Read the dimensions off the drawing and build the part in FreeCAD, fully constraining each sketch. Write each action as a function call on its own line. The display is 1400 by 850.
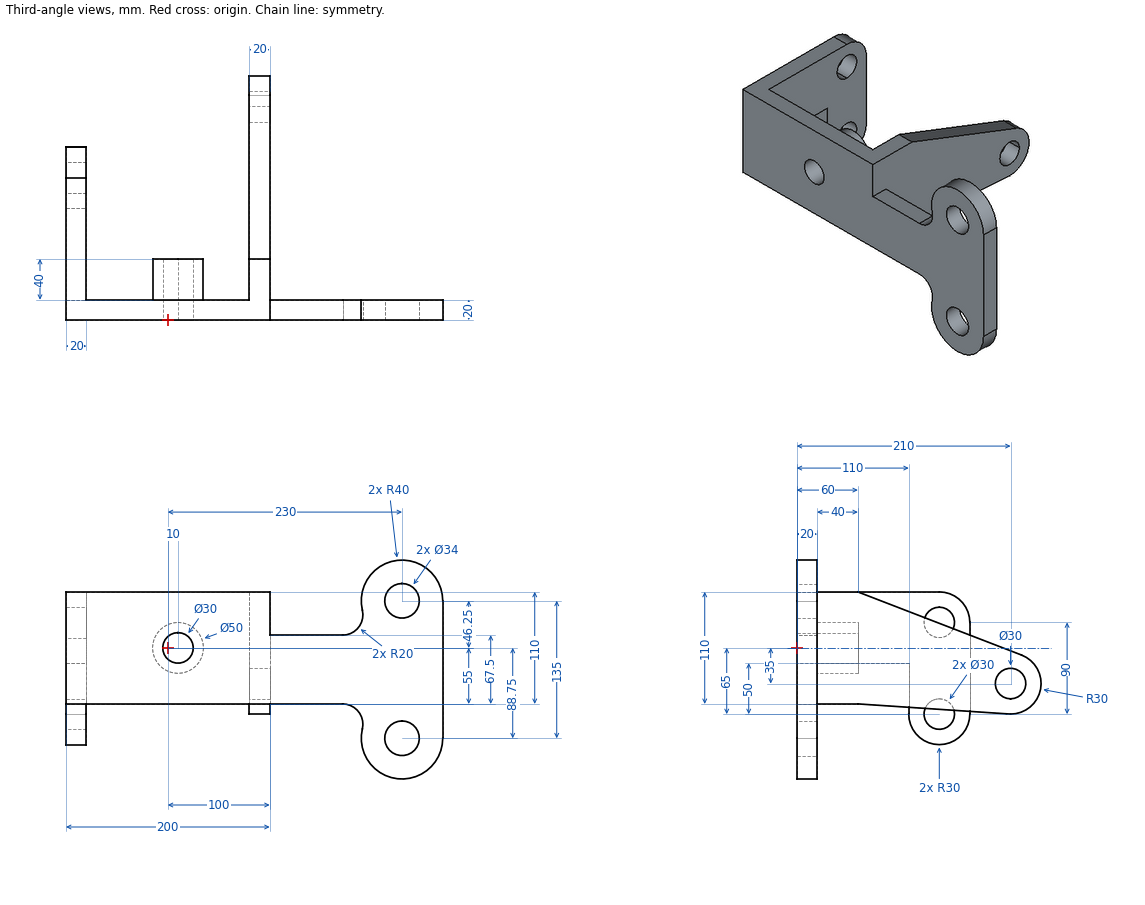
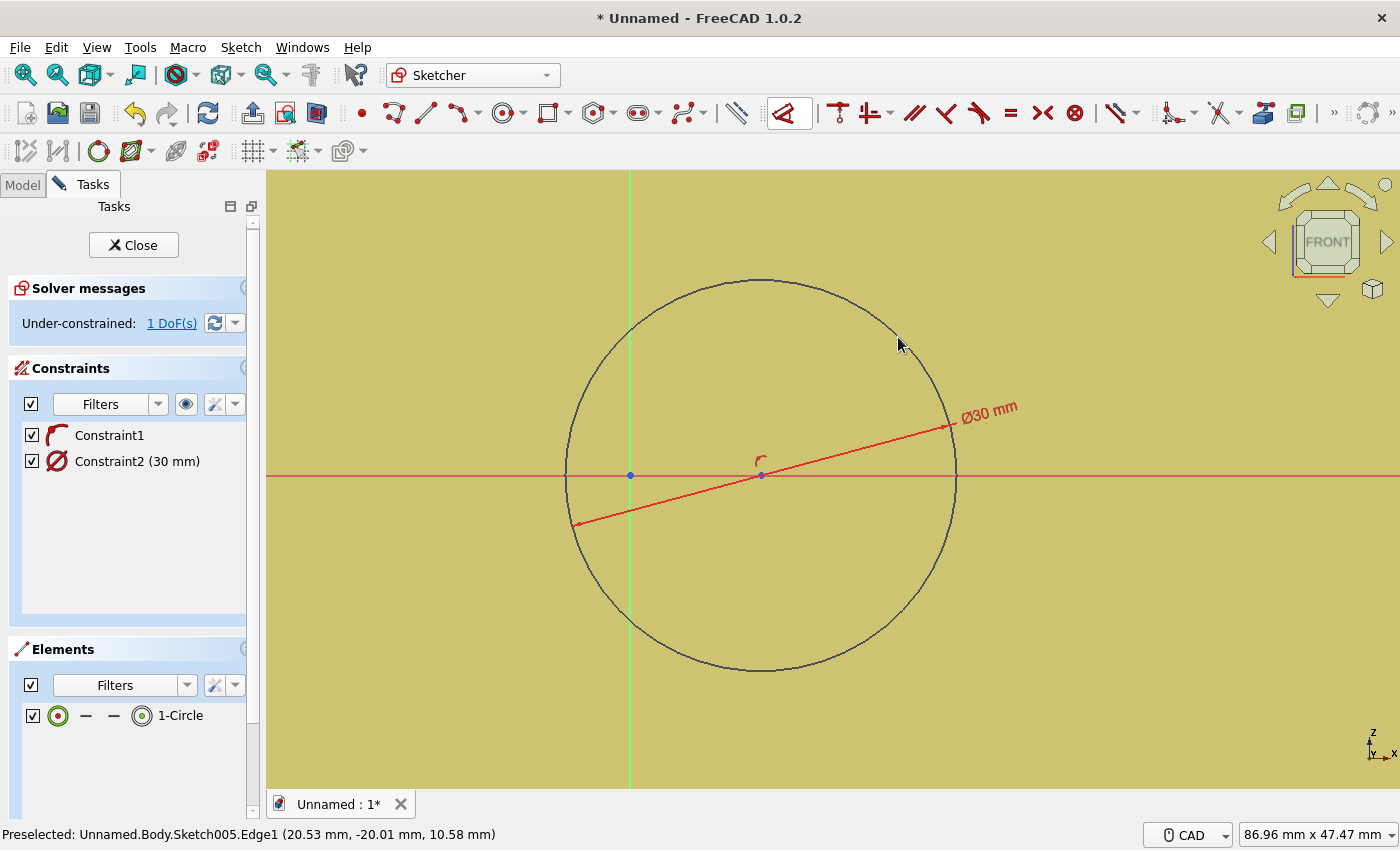
click(761, 476)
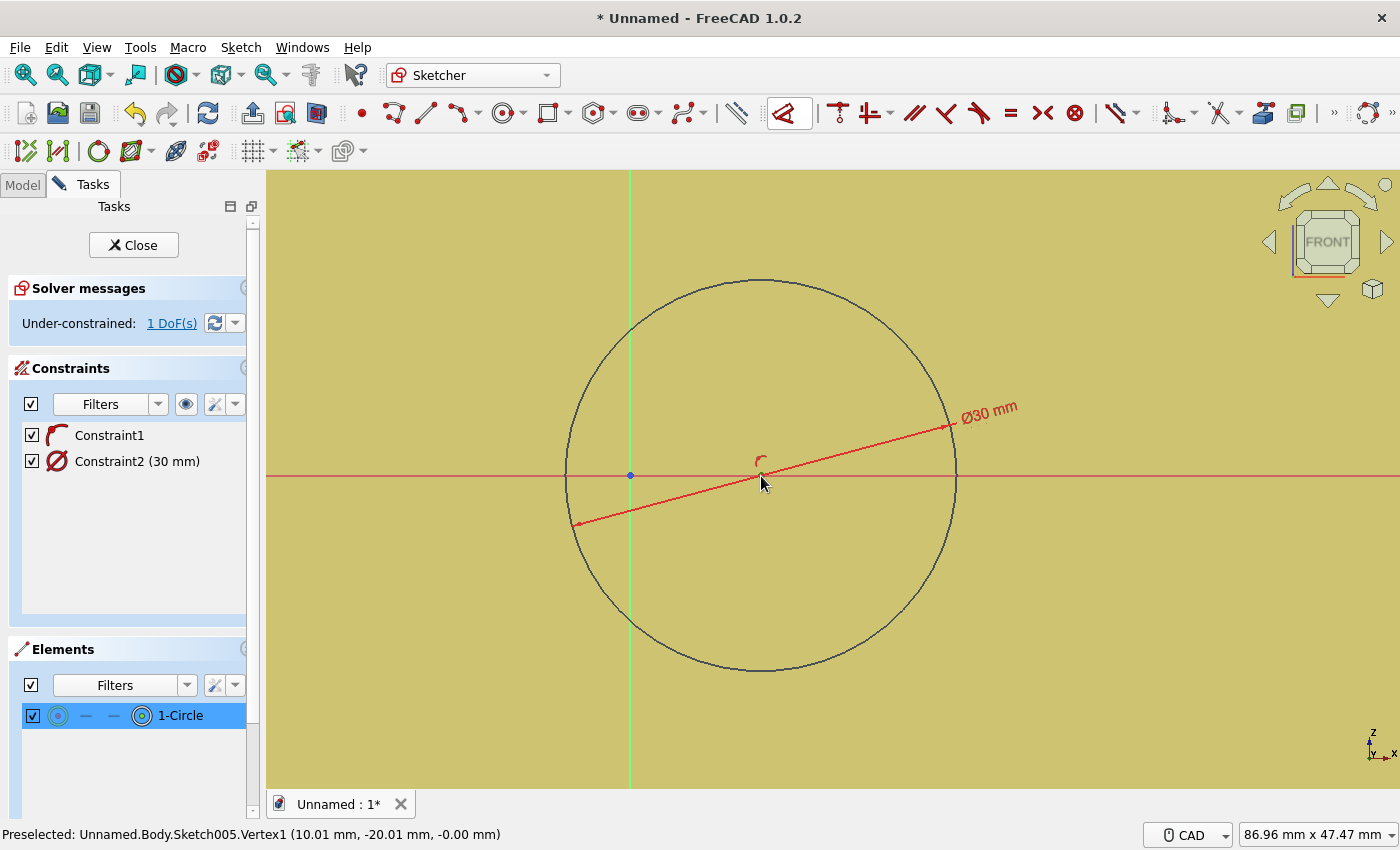
click(806, 114)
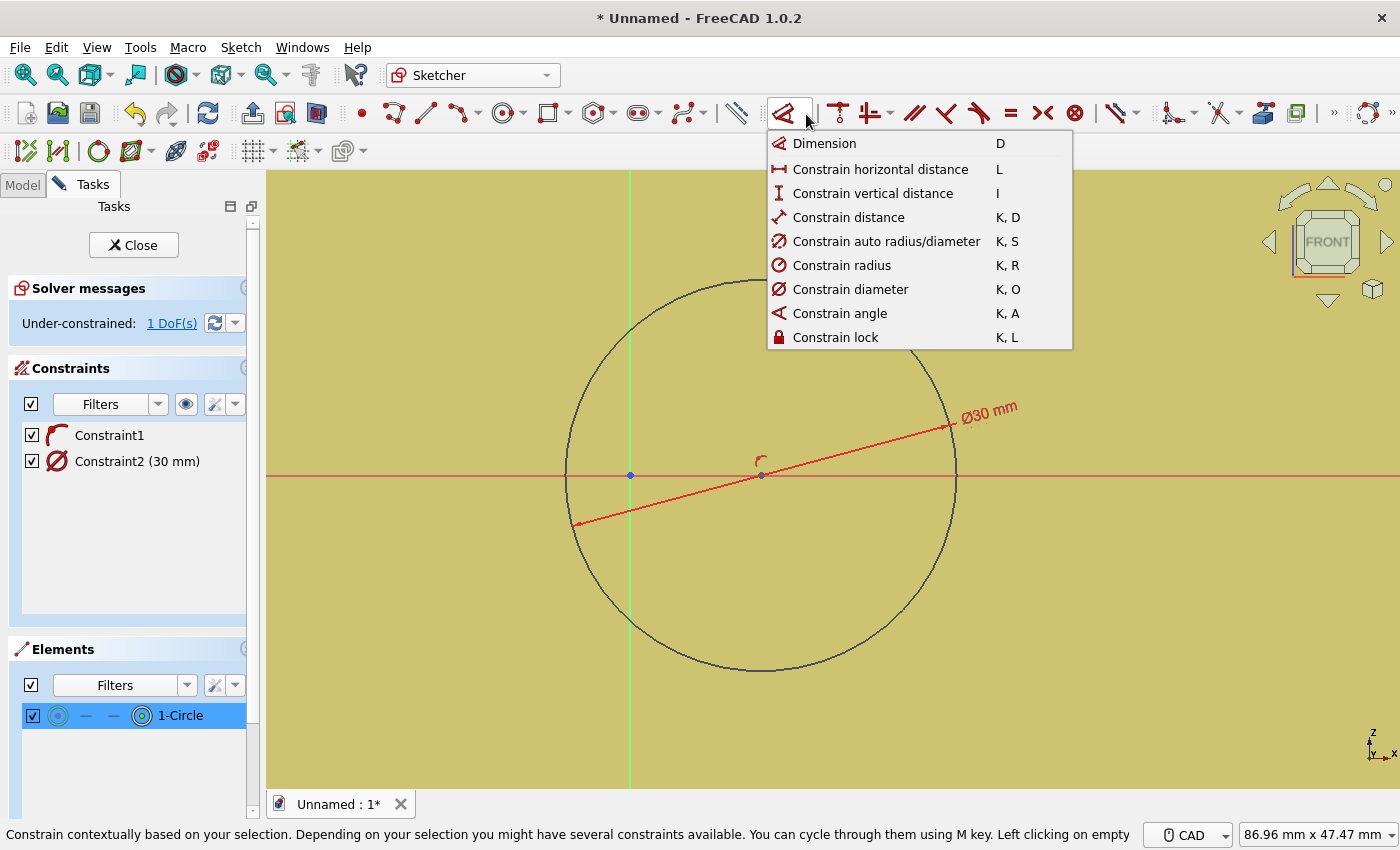
click(920, 169)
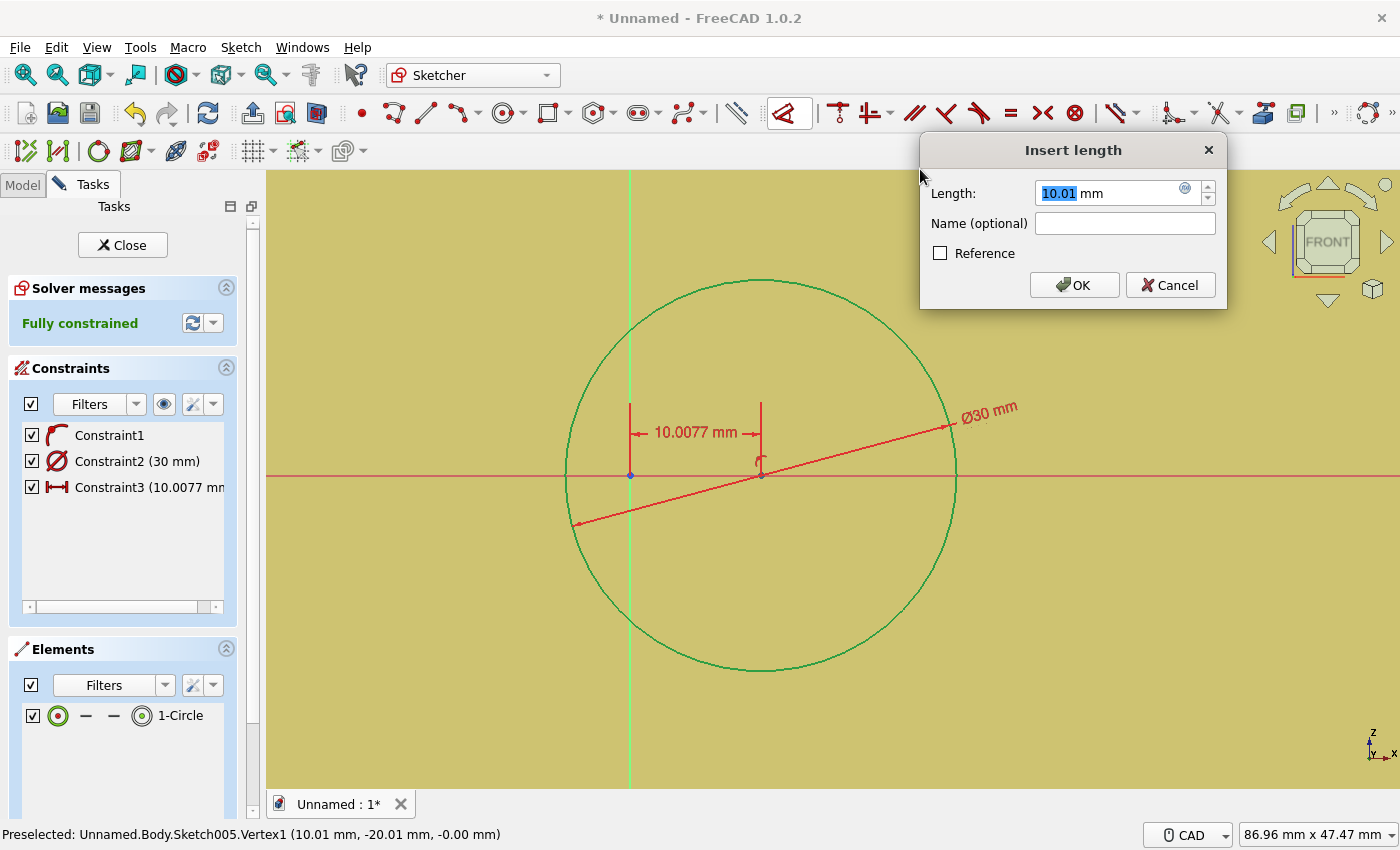
text(10)
key(Return)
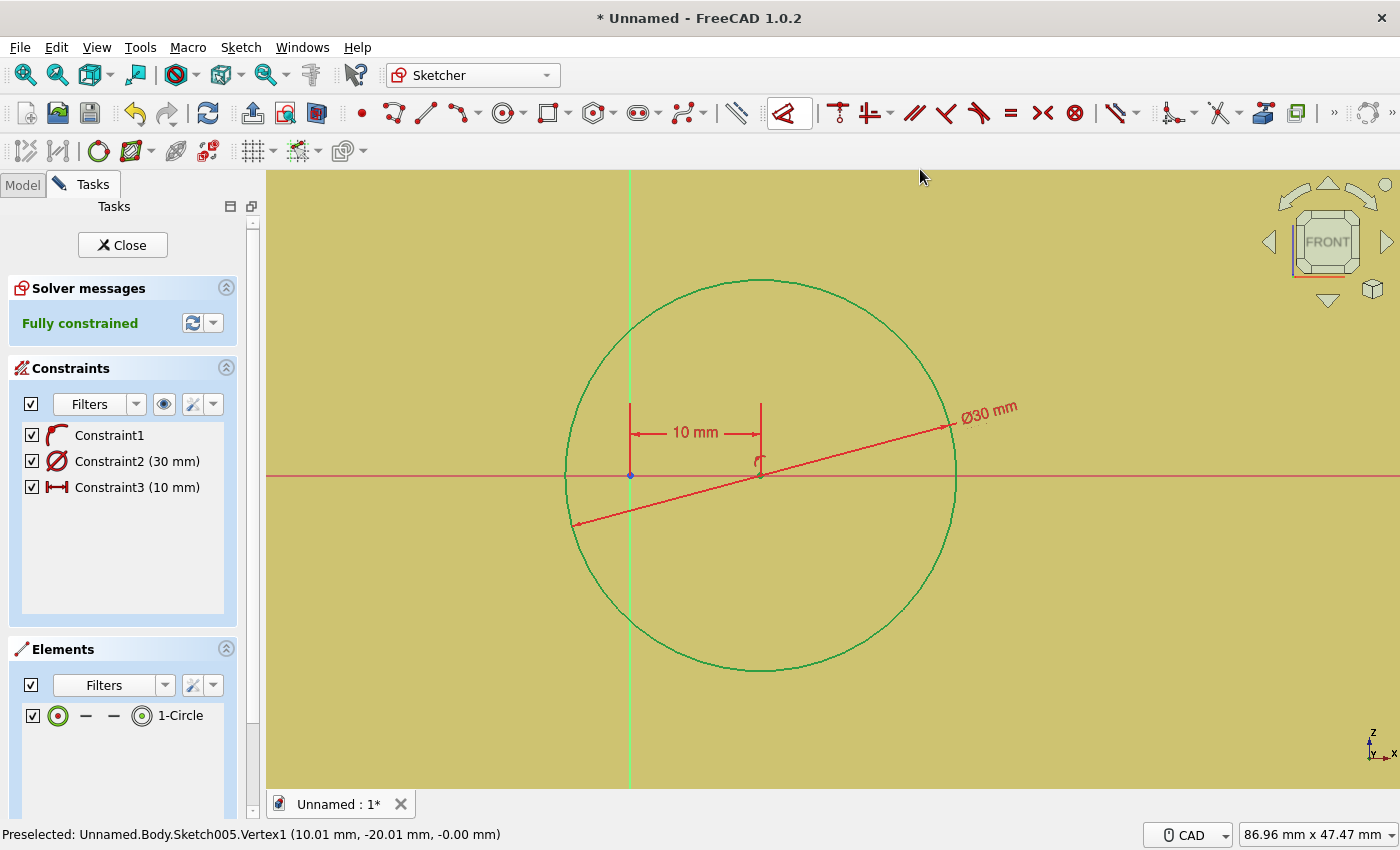
click(123, 245)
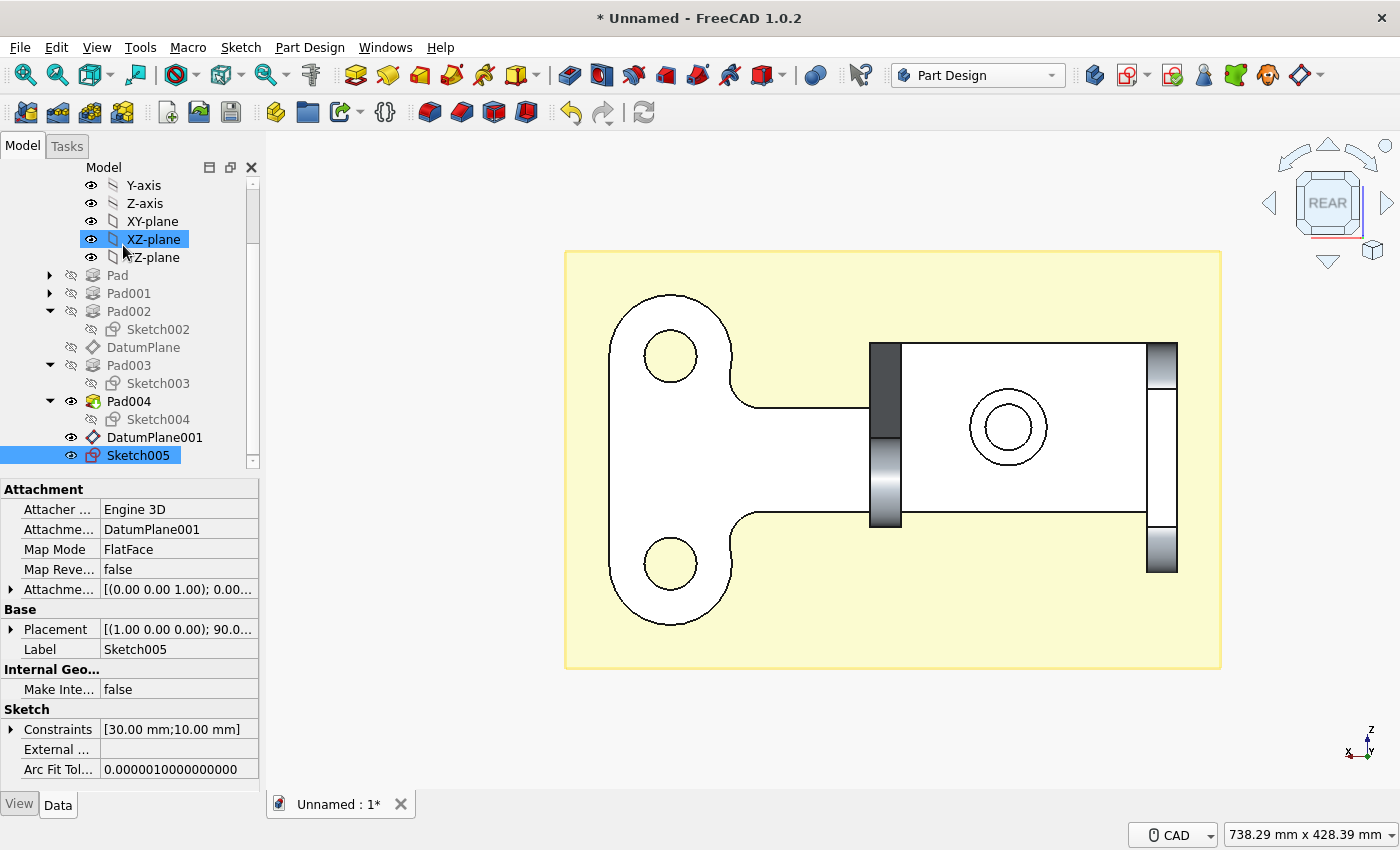
click(570, 76)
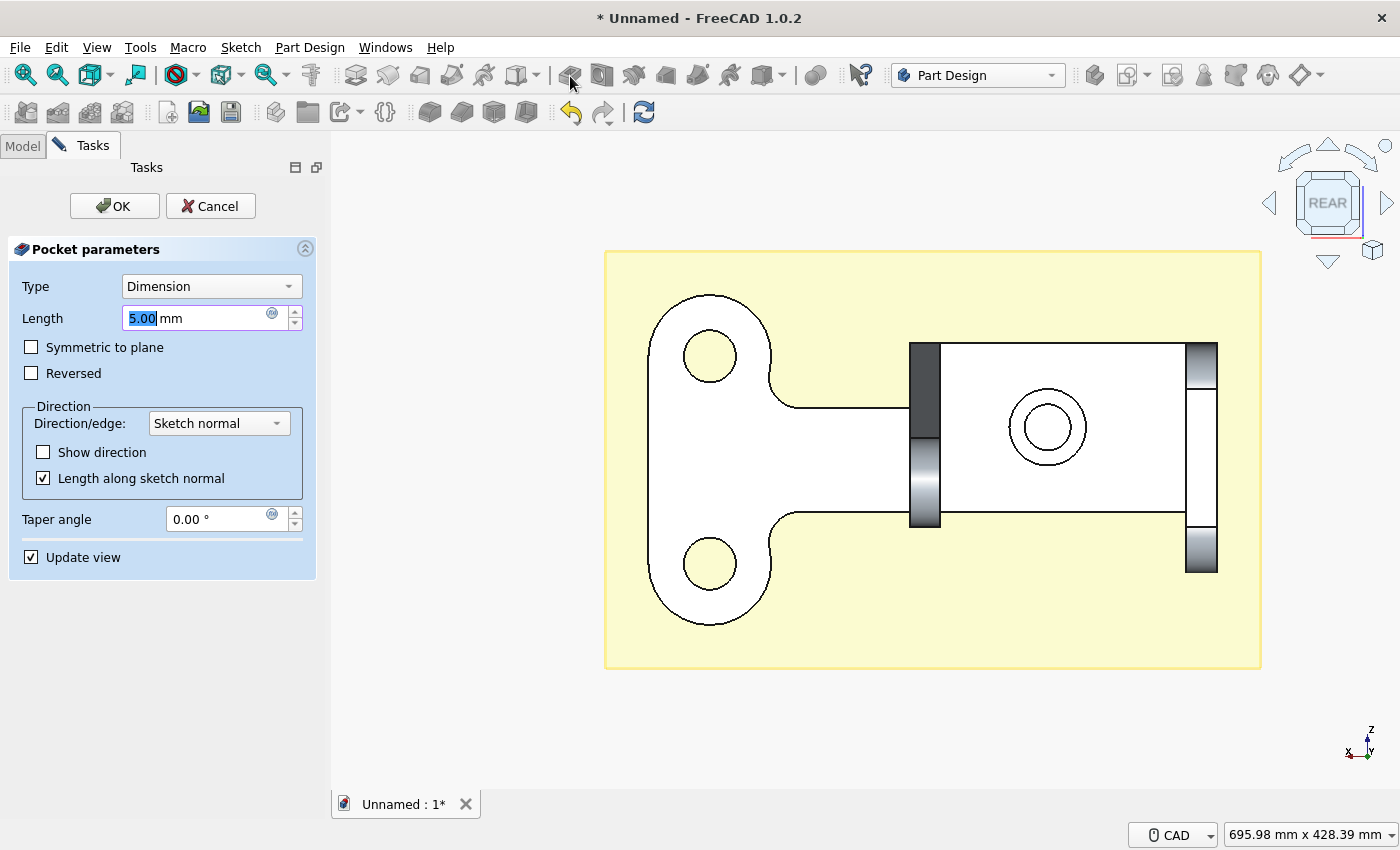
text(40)
key(Tab)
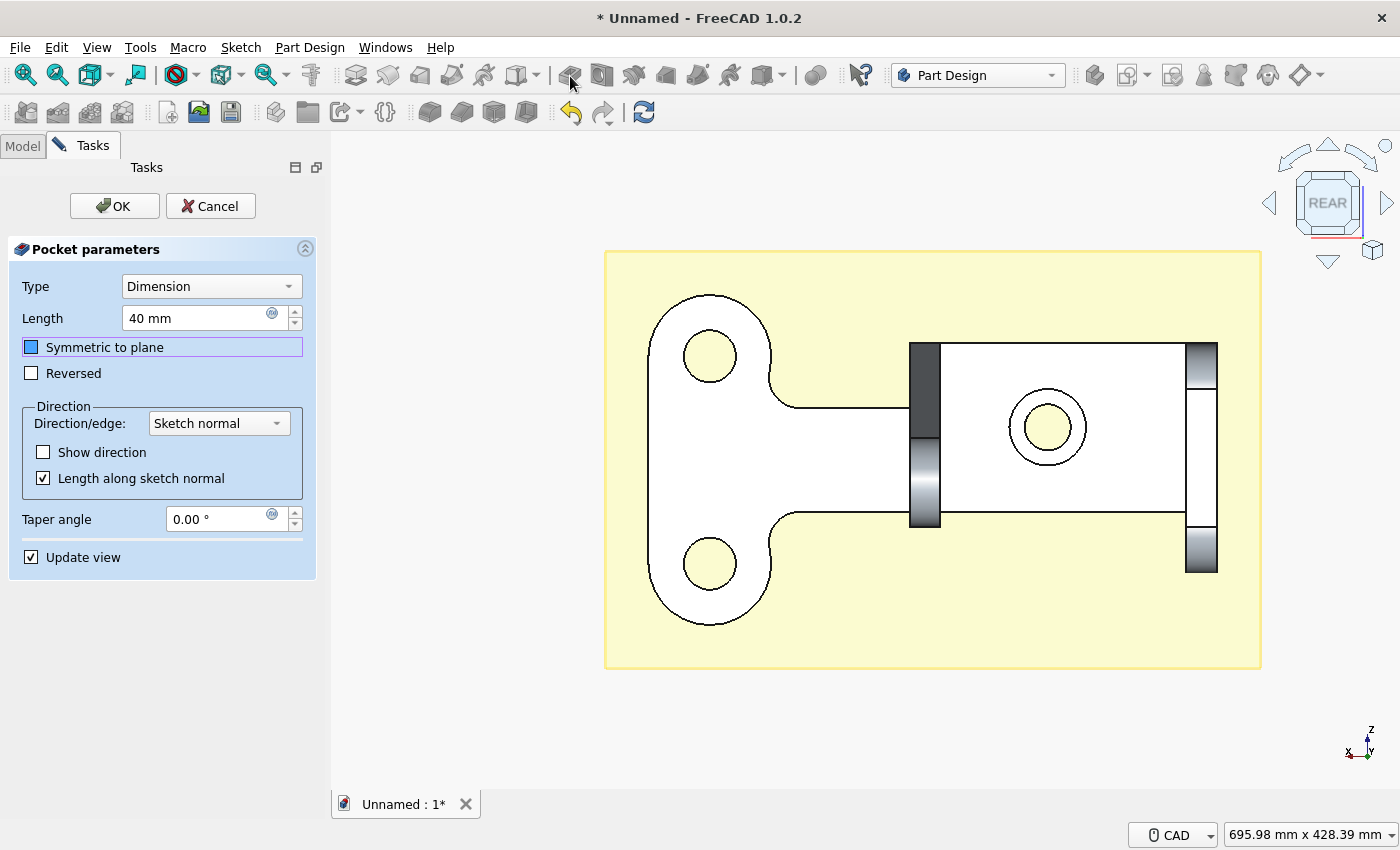
click(115, 206)